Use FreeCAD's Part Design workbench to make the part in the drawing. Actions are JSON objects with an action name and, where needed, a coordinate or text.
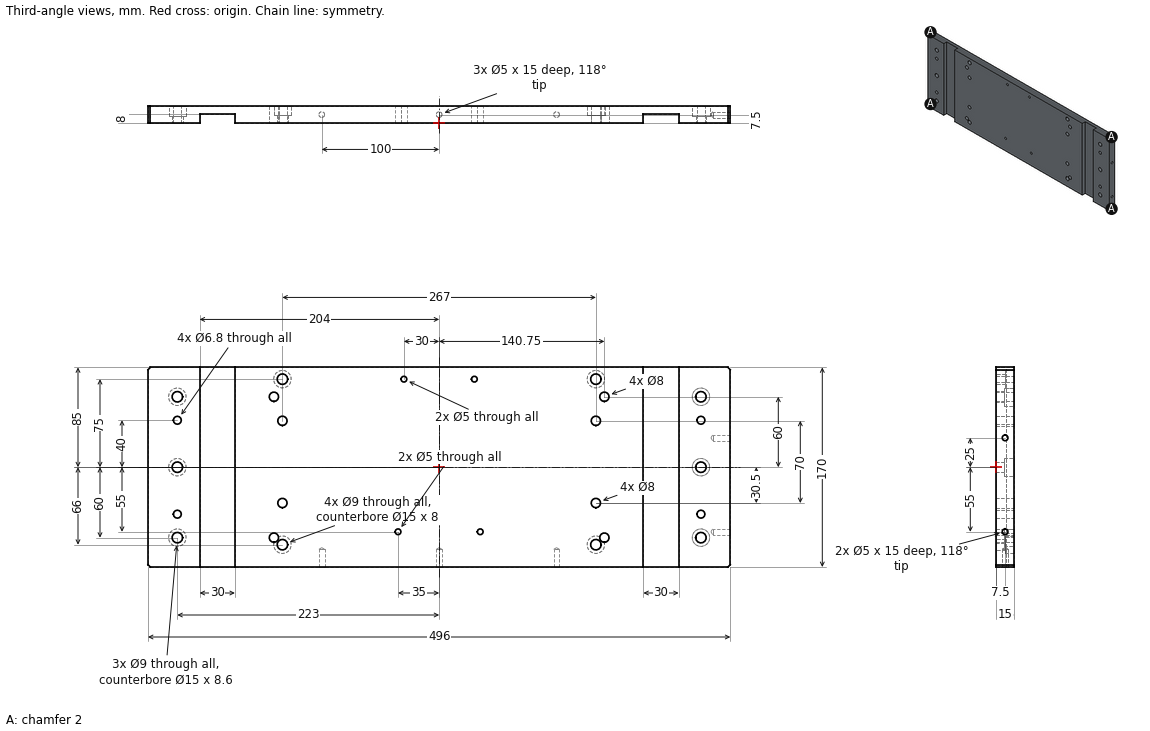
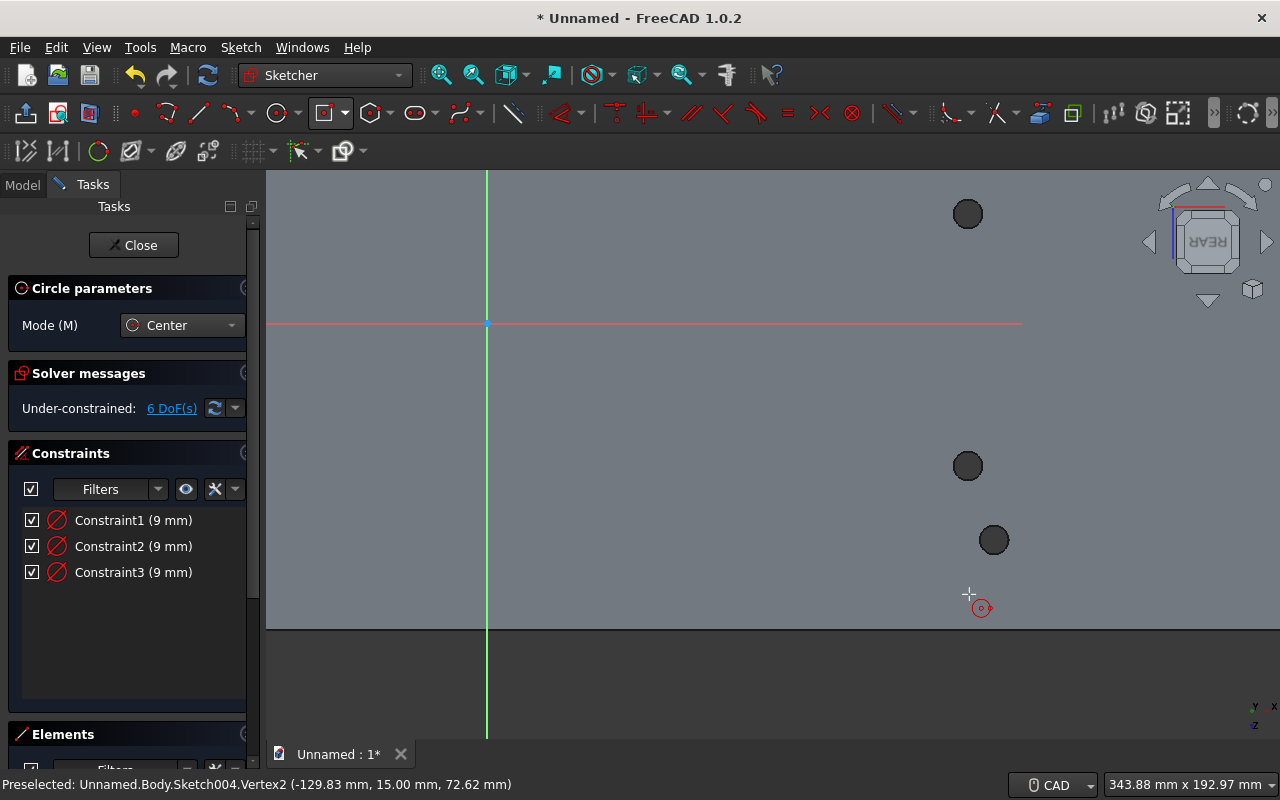
{"action": "left_click", "coordinate": [967, 594]}
{"action": "mouse_move", "coordinate": [984, 576]}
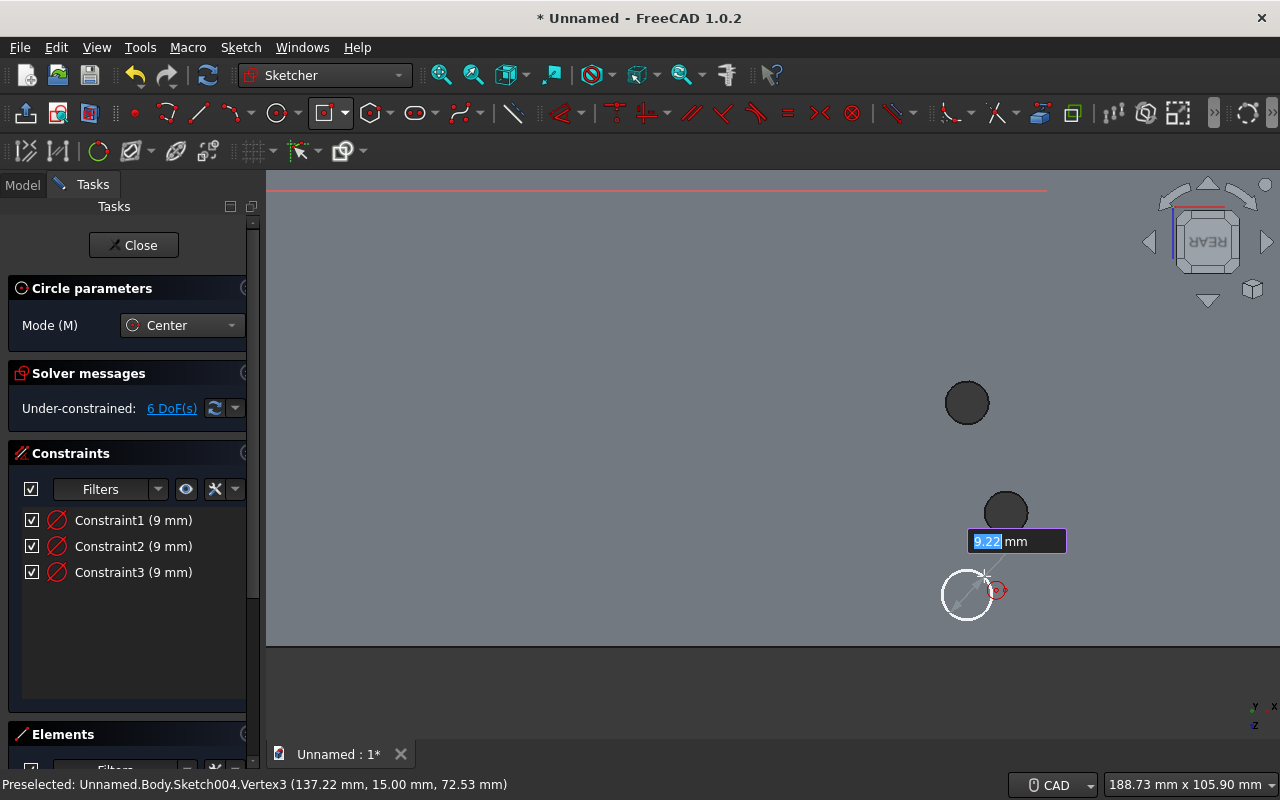
{"action": "type", "text": "9"}
{"action": "key", "text": "Return"}
{"action": "key", "text": "Escape"}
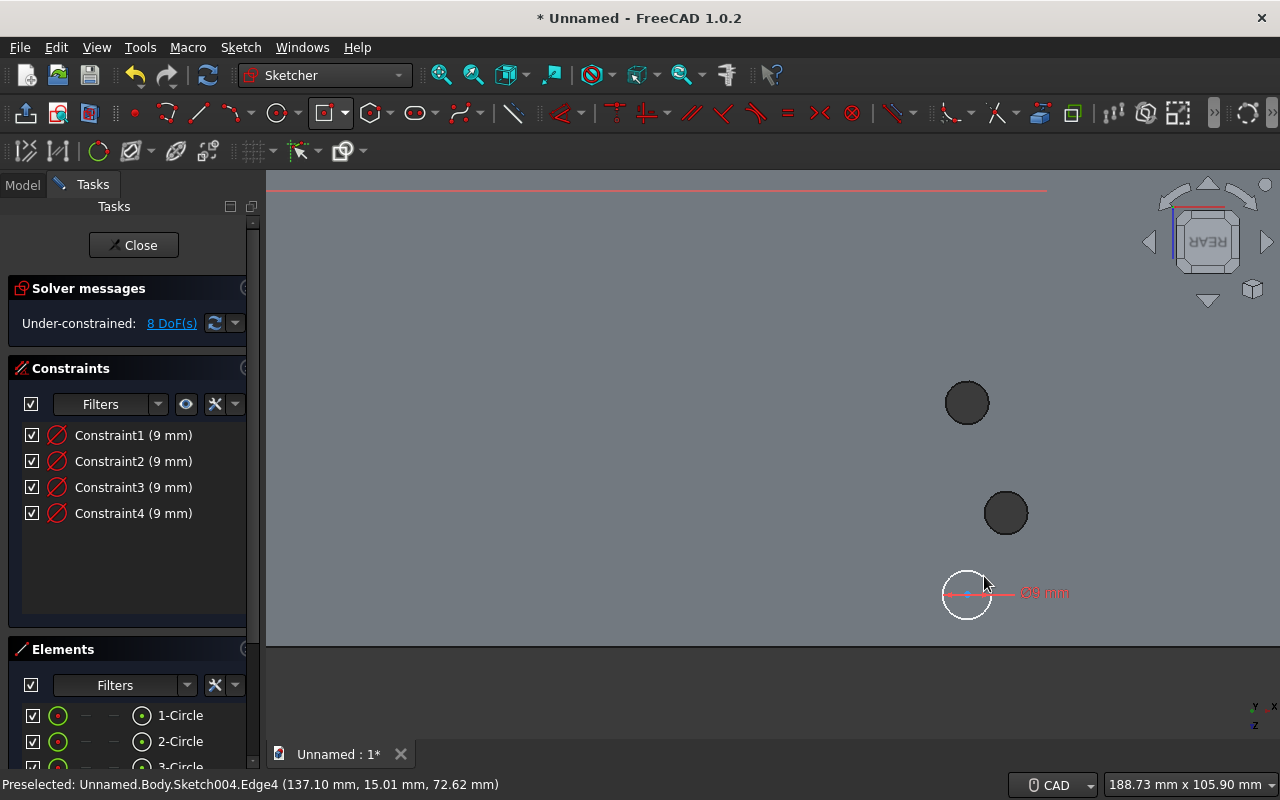
{"action": "scroll", "coordinate": [969, 594], "scroll_direction": "down", "scroll_amount": 5}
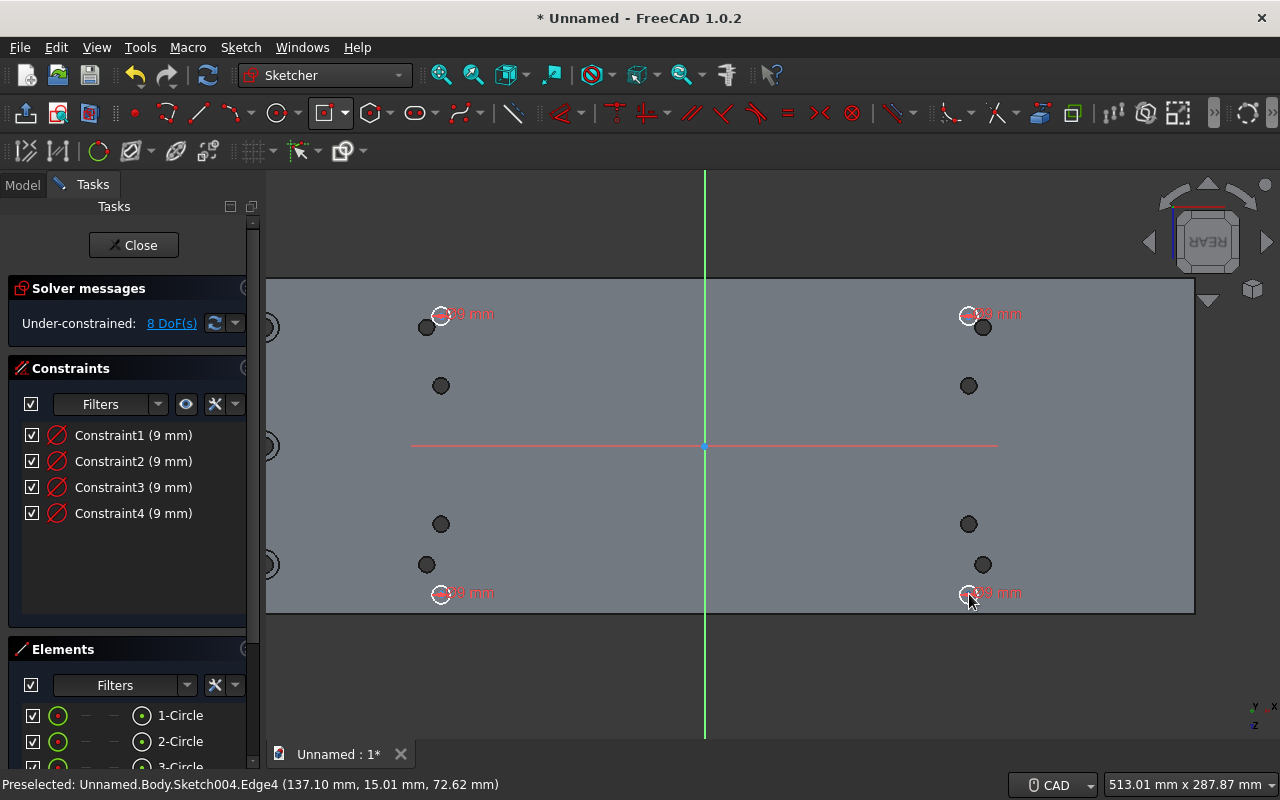
{"action": "left_click", "coordinate": [441, 316]}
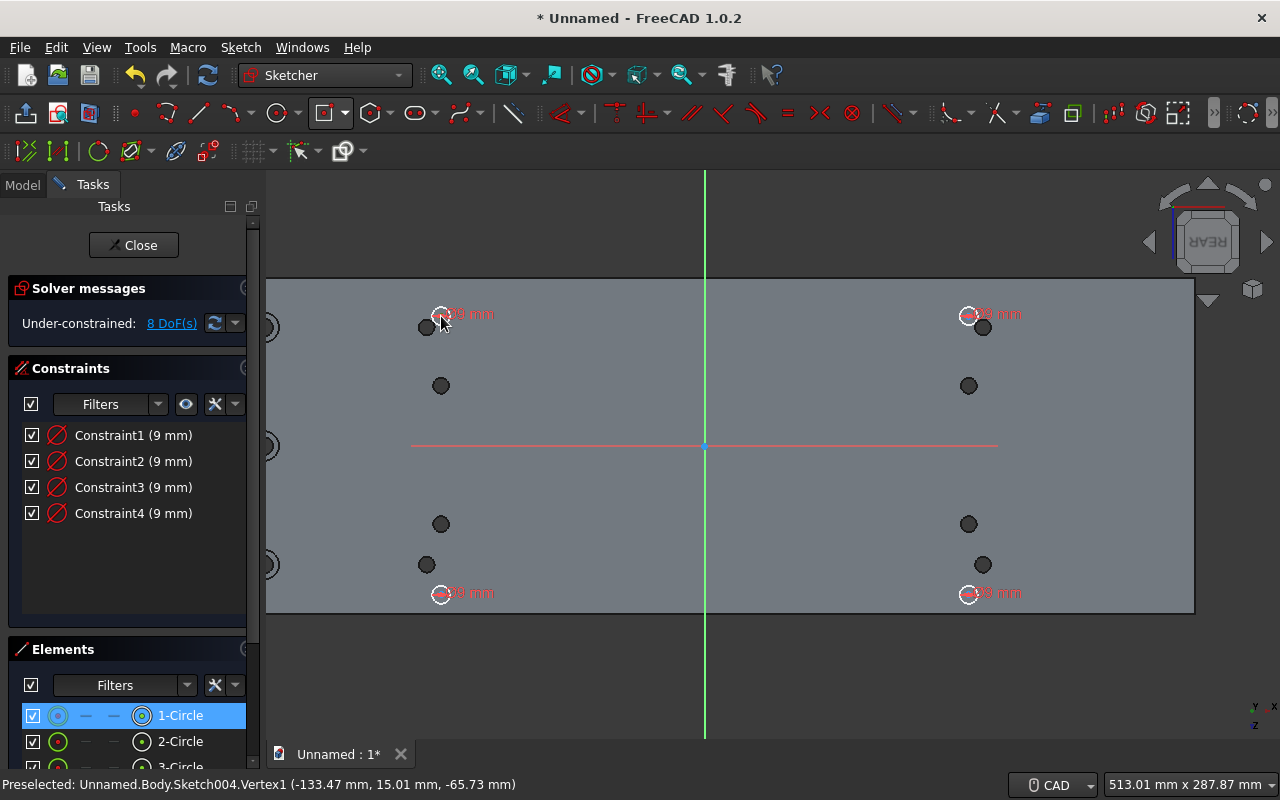
{"action": "left_click", "coordinate": [969, 316]}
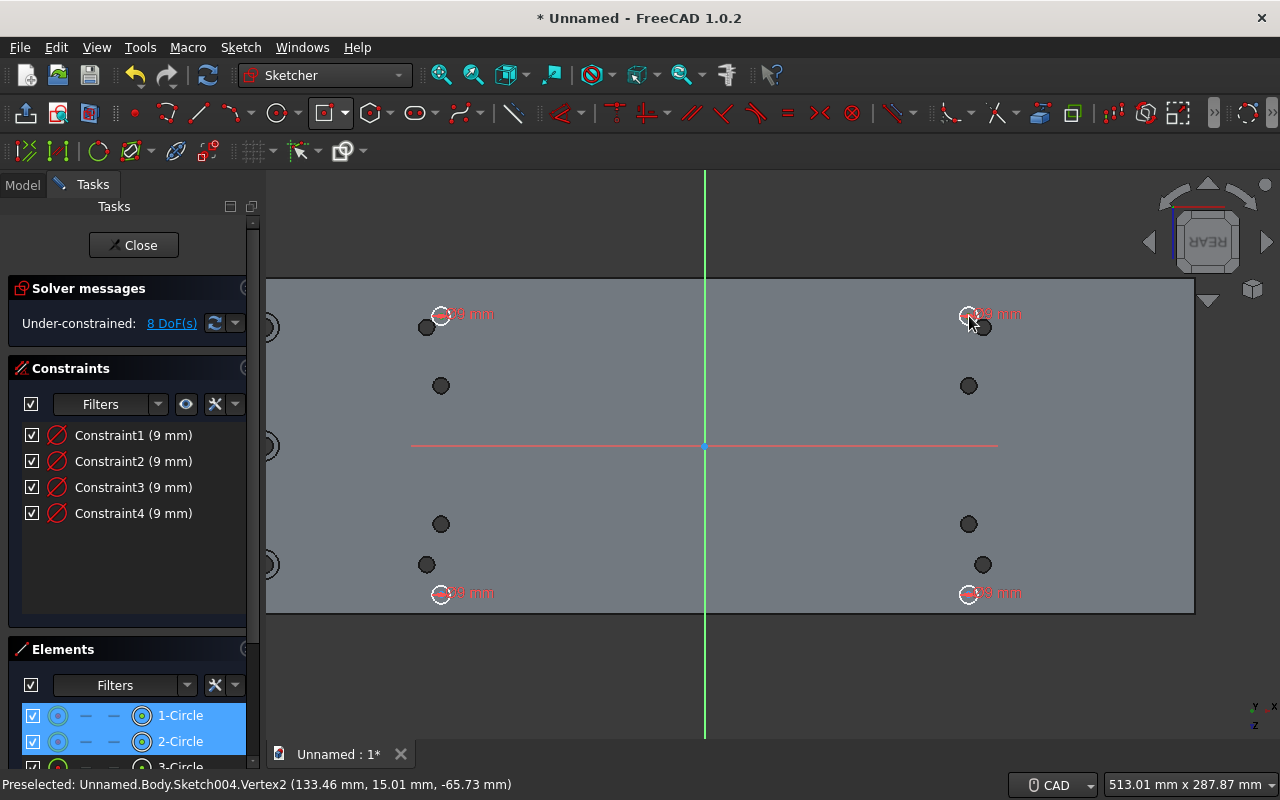
{"action": "left_click", "coordinate": [705, 674]}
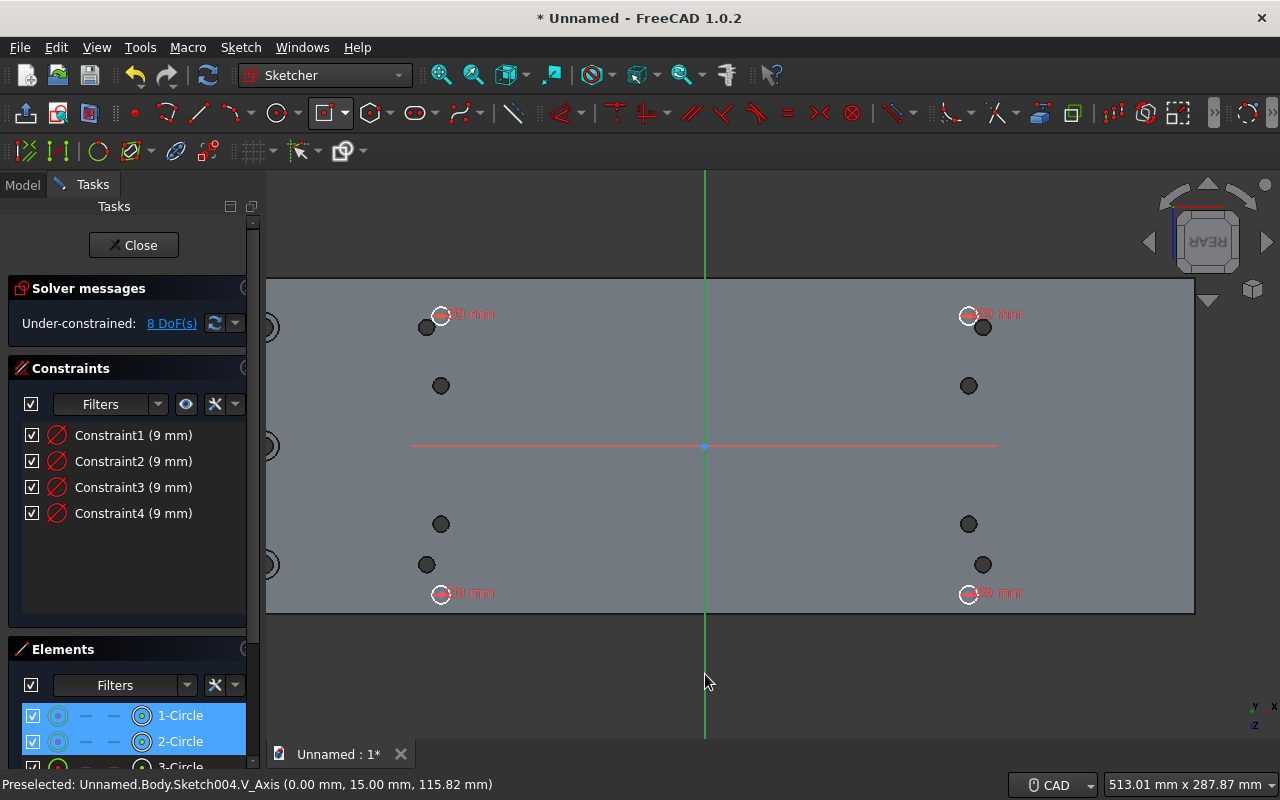
{"action": "left_click", "coordinate": [820, 114]}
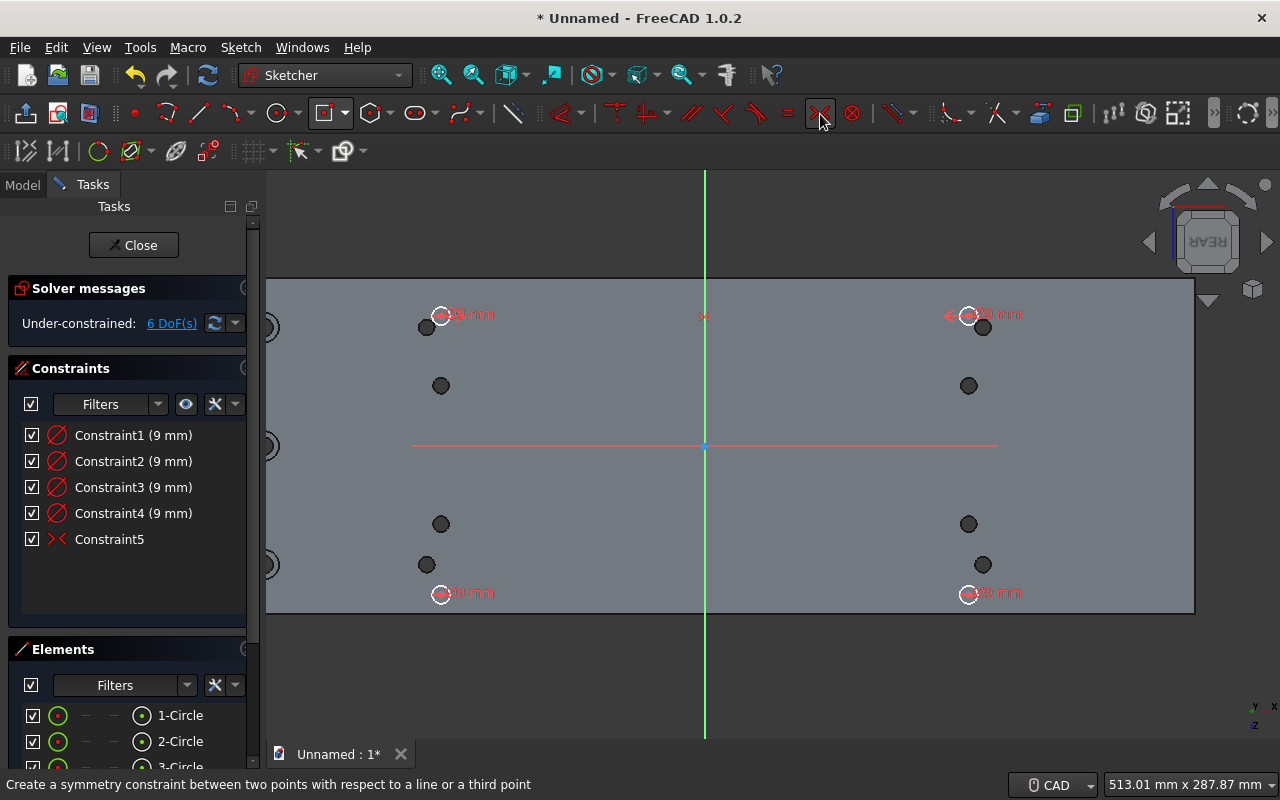
{"action": "left_click", "coordinate": [441, 595]}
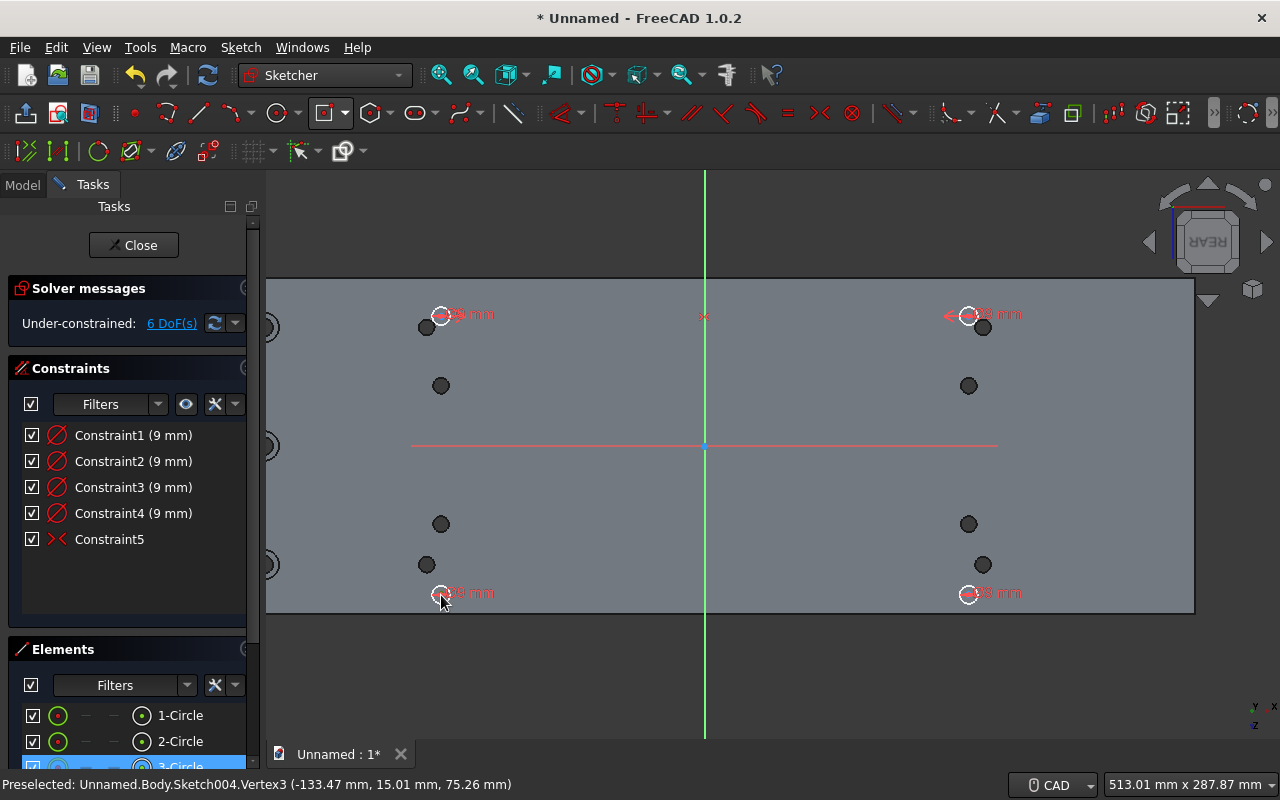
{"action": "left_click", "coordinate": [969, 595]}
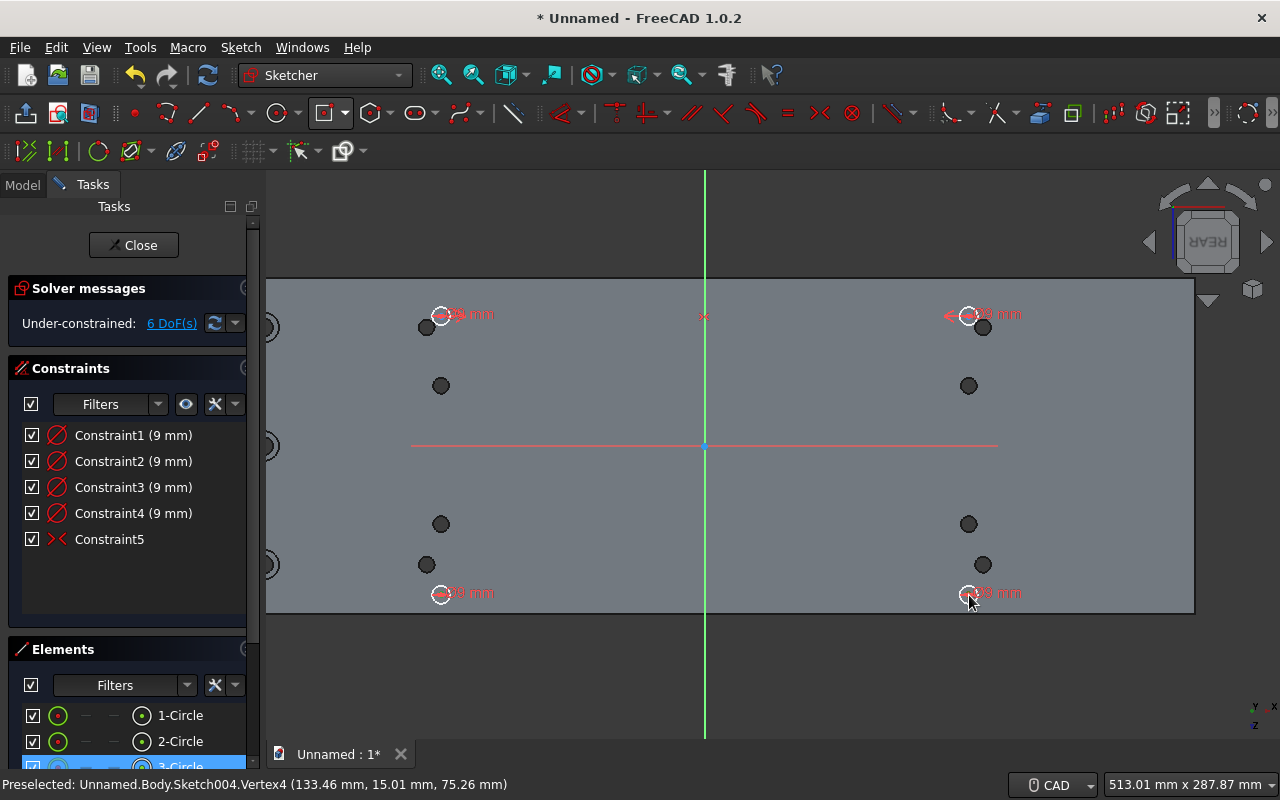
{"action": "left_click", "coordinate": [705, 674]}